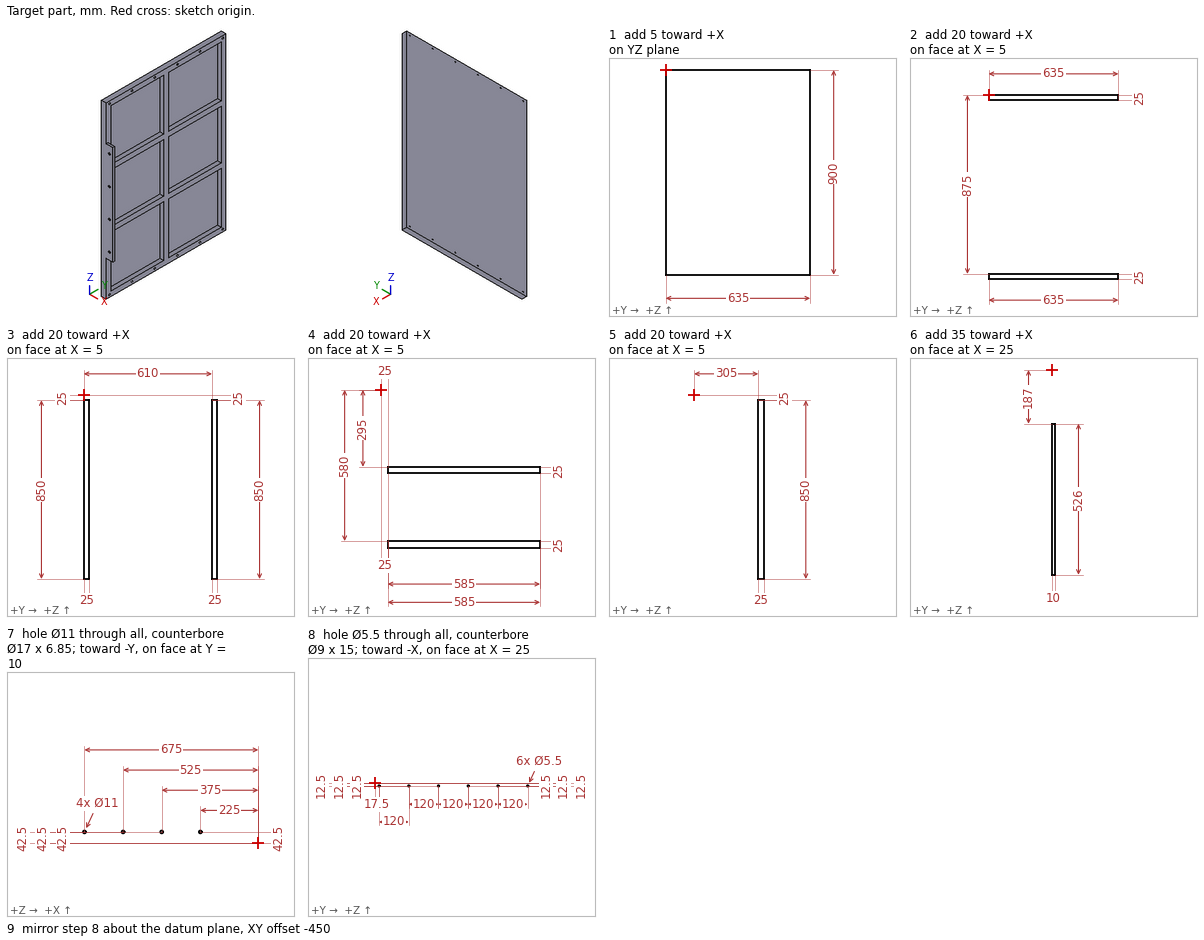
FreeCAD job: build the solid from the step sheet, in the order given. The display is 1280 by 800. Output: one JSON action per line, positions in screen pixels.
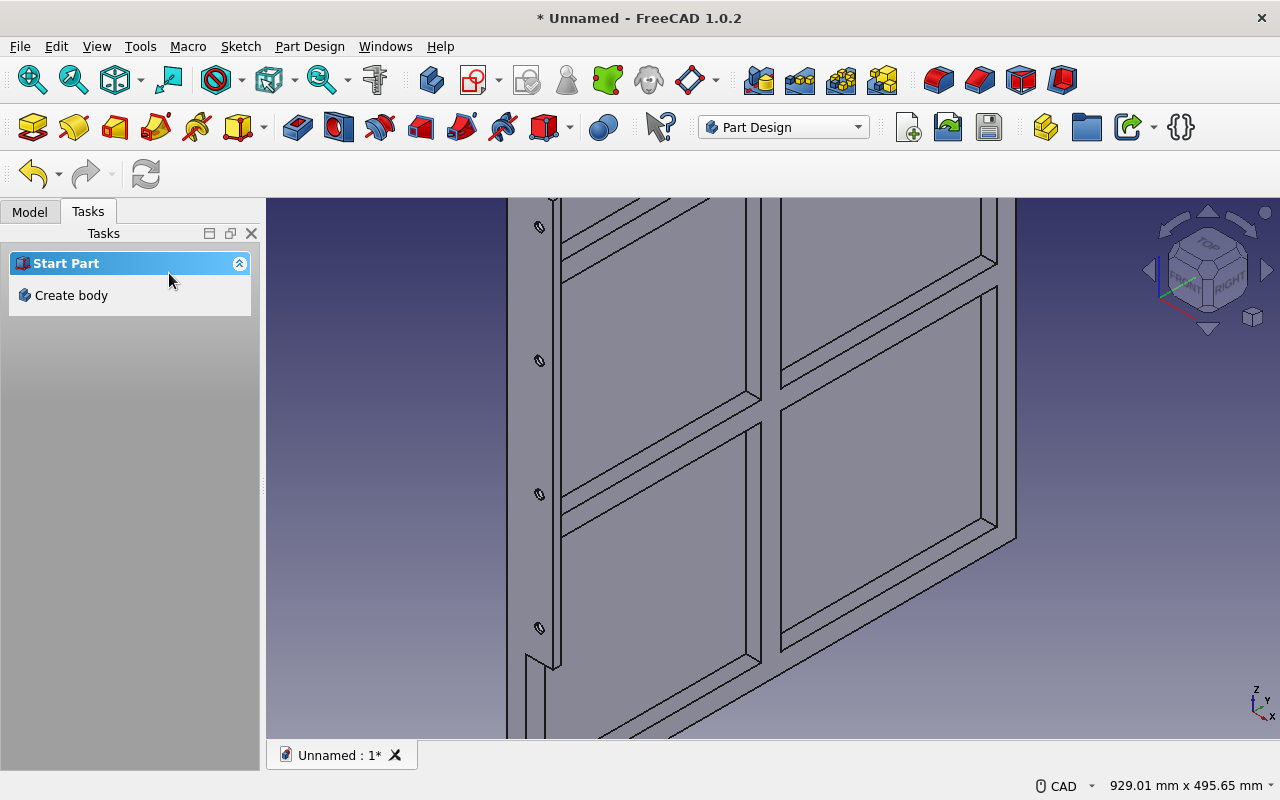
{"action": "left_click", "coordinate": [33, 80]}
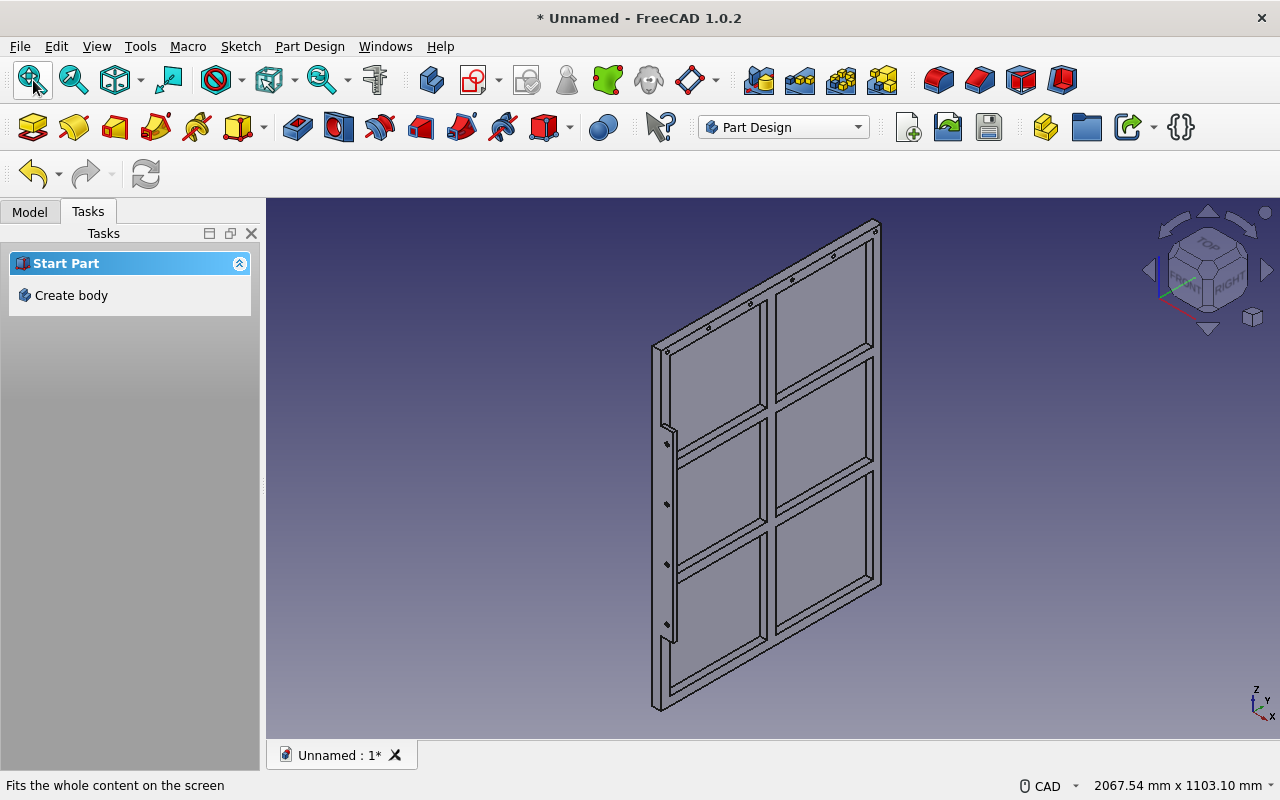
{"action": "left_click", "coordinate": [30, 212]}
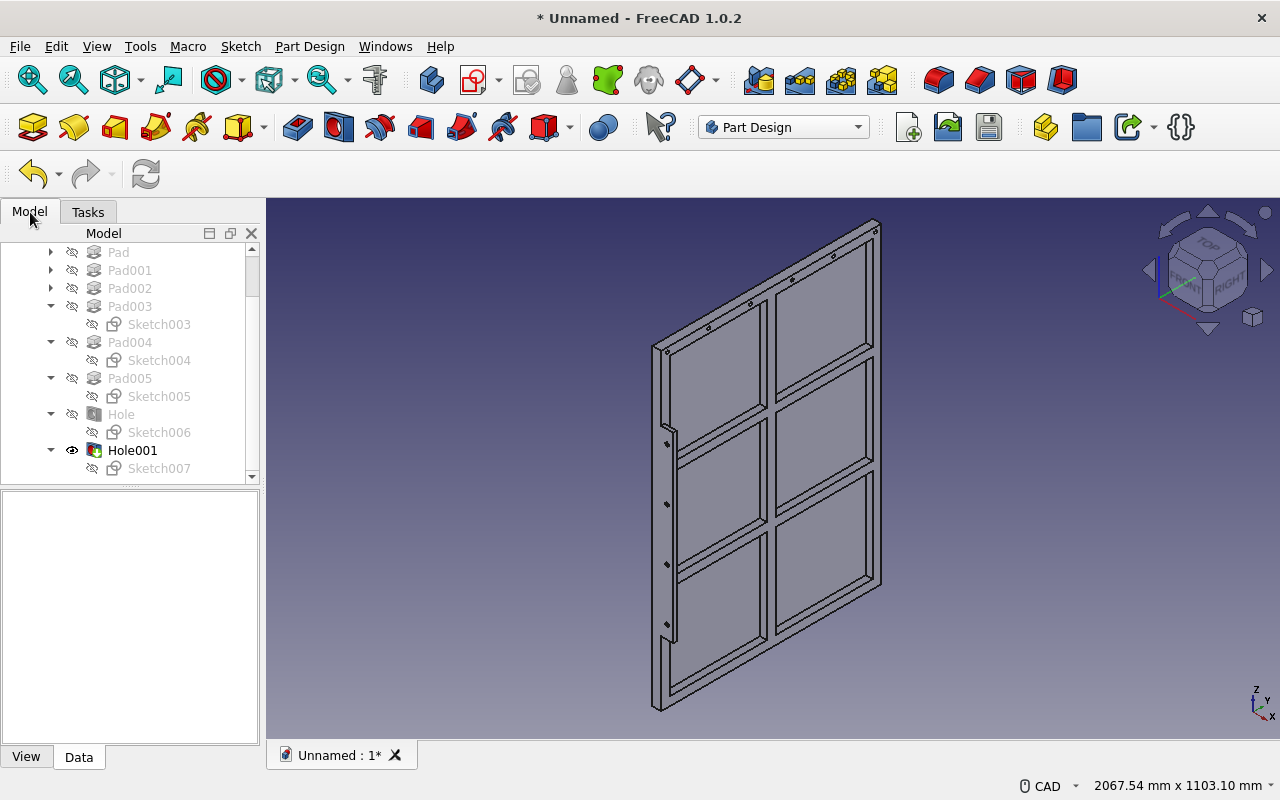
{"action": "scroll", "coordinate": [141, 356], "scroll_direction": "down", "scroll_amount": 3}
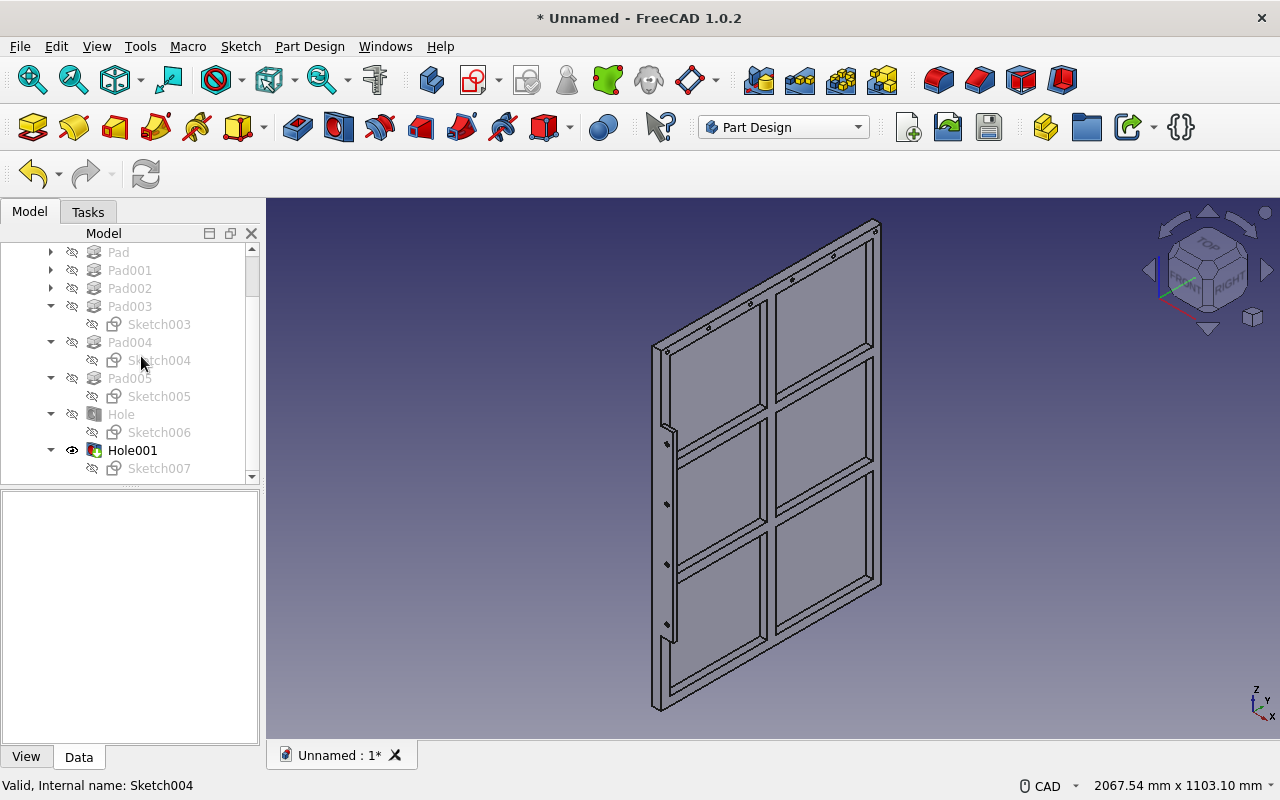
{"action": "scroll", "coordinate": [141, 356], "scroll_direction": "up", "scroll_amount": 15}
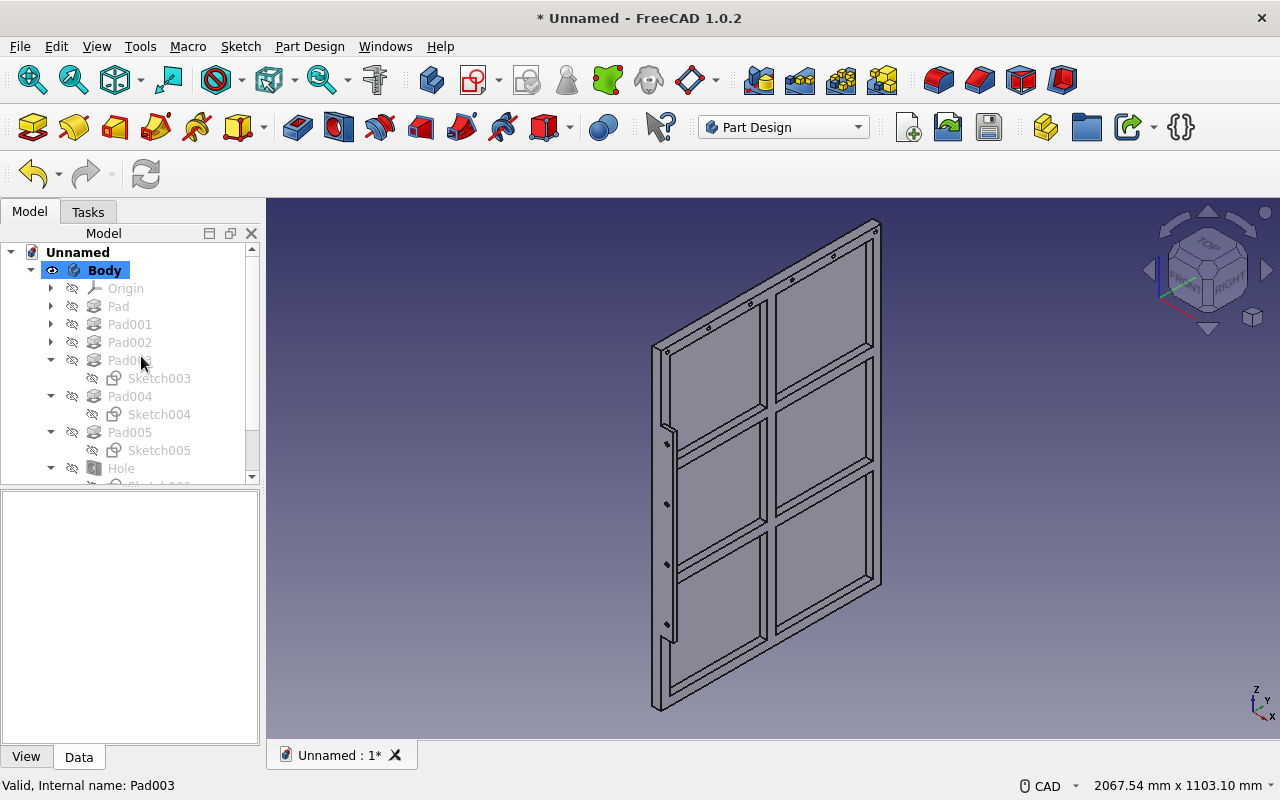
{"action": "left_click", "coordinate": [51, 288]}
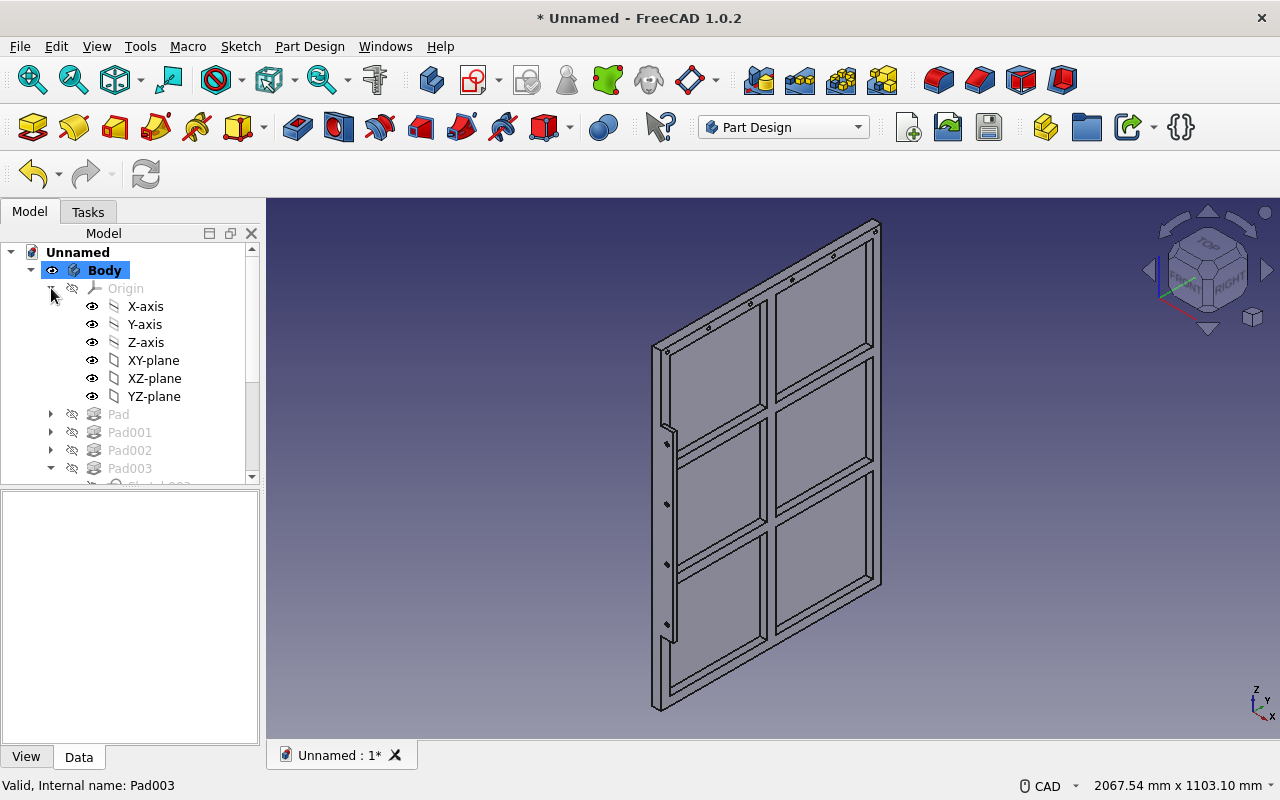
{"action": "left_click", "coordinate": [137, 360]}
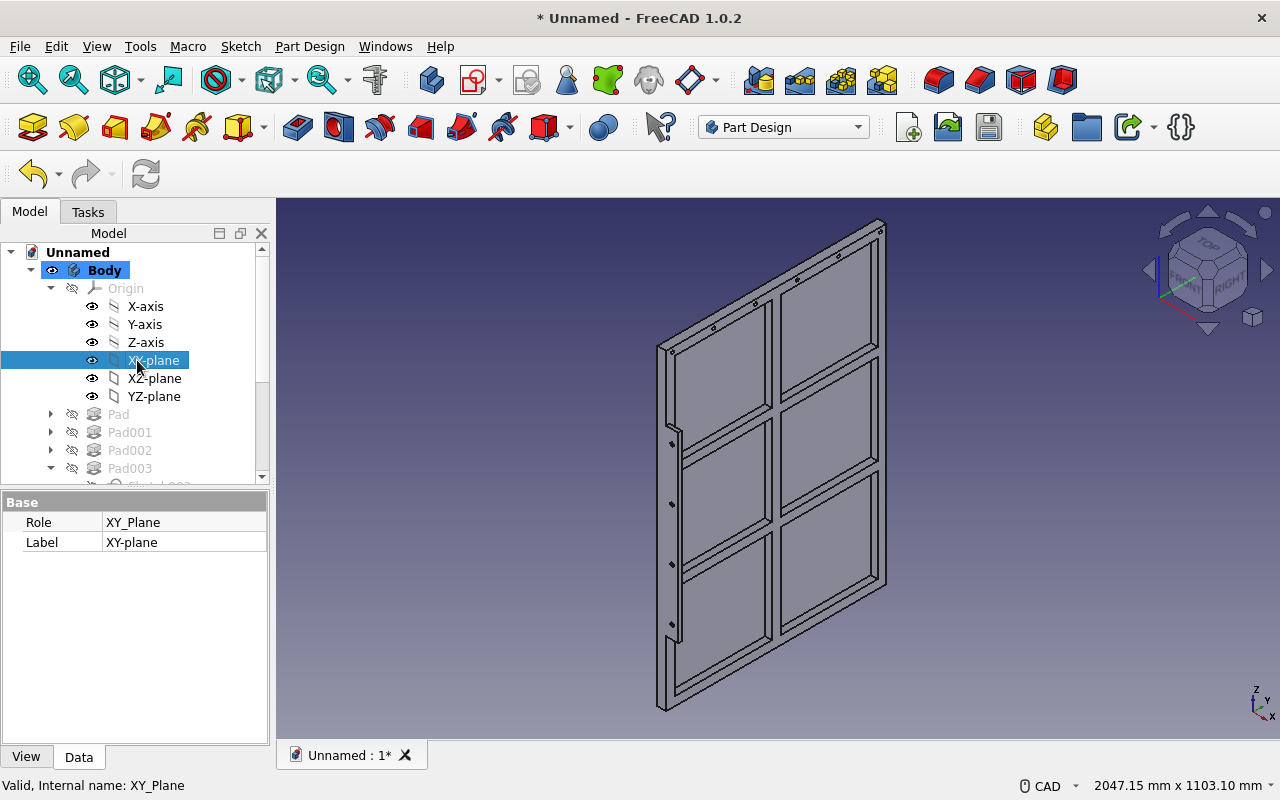
{"action": "left_click", "coordinate": [690, 80]}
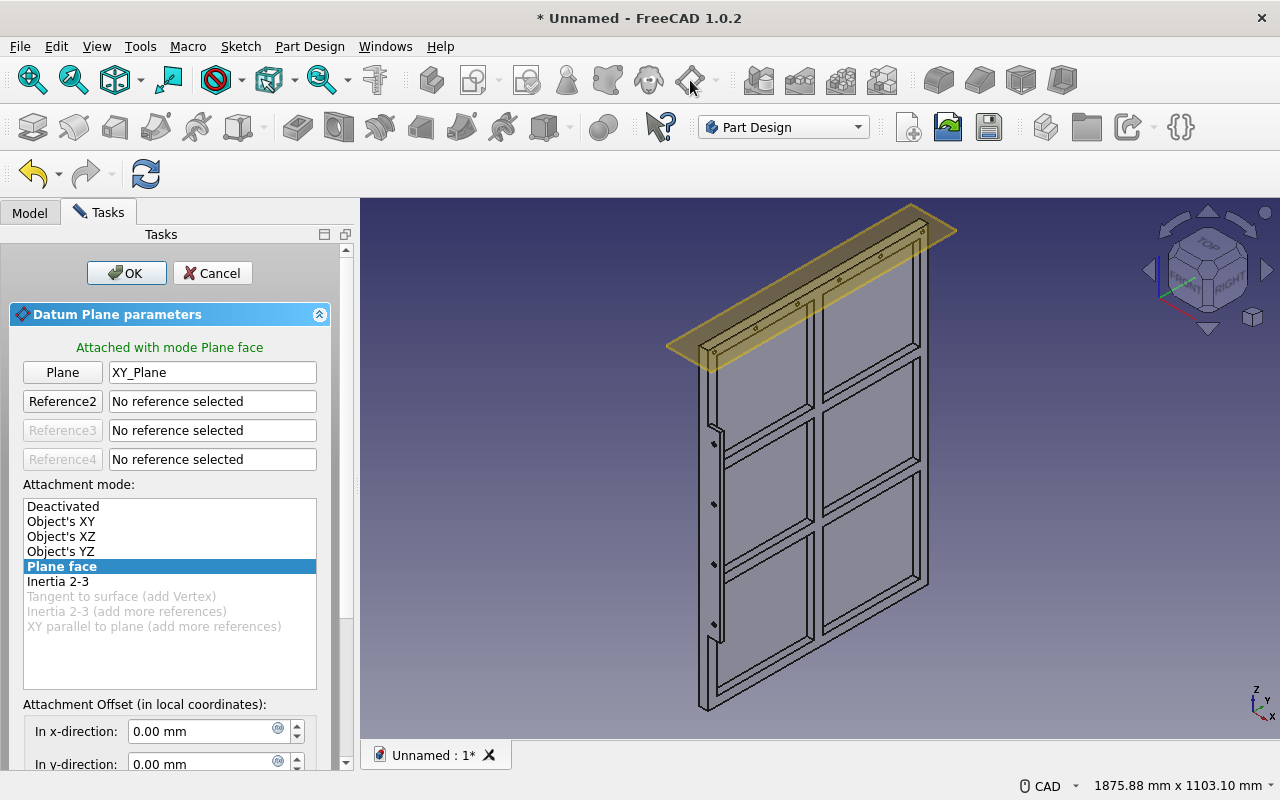
{"action": "scroll", "coordinate": [346, 507], "scroll_direction": "down", "scroll_amount": 2}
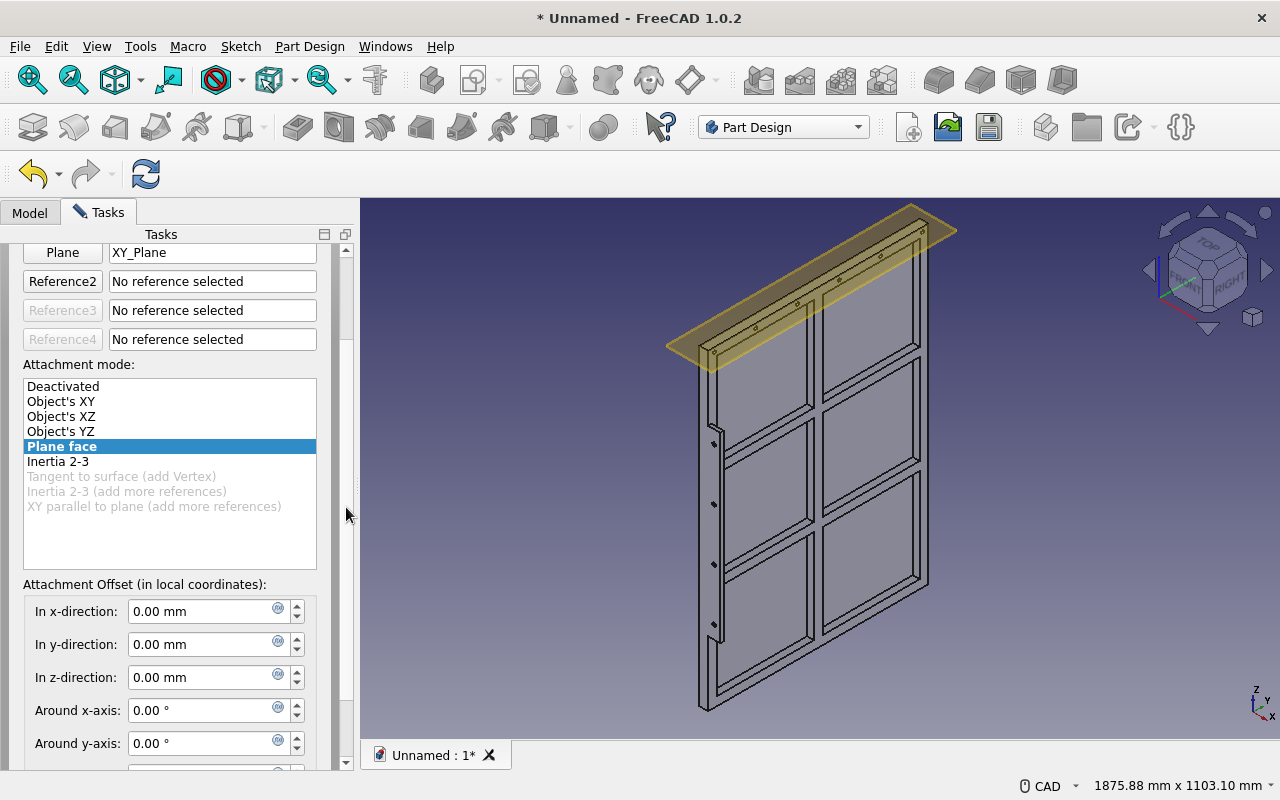
{"action": "triple_click", "coordinate": [210, 678]}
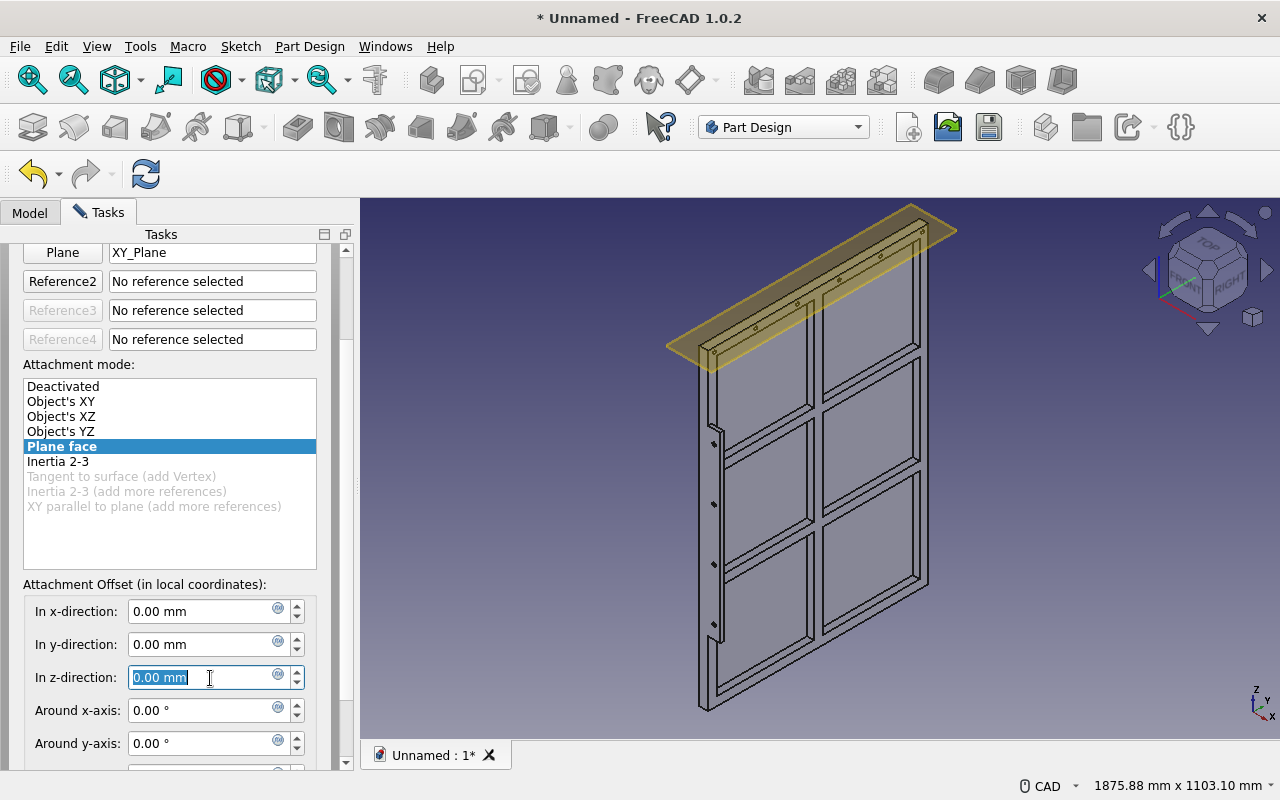
{"action": "type", "text": "-450"}
{"action": "key", "text": "Tab"}